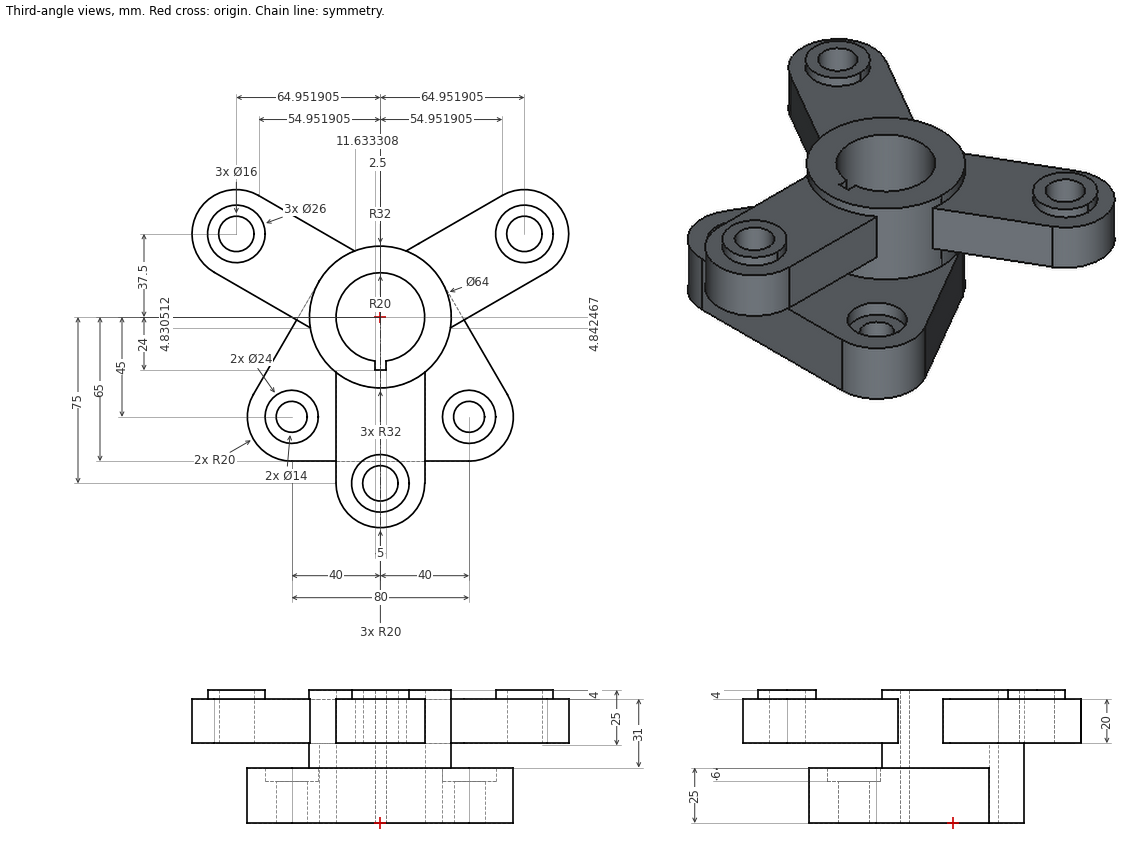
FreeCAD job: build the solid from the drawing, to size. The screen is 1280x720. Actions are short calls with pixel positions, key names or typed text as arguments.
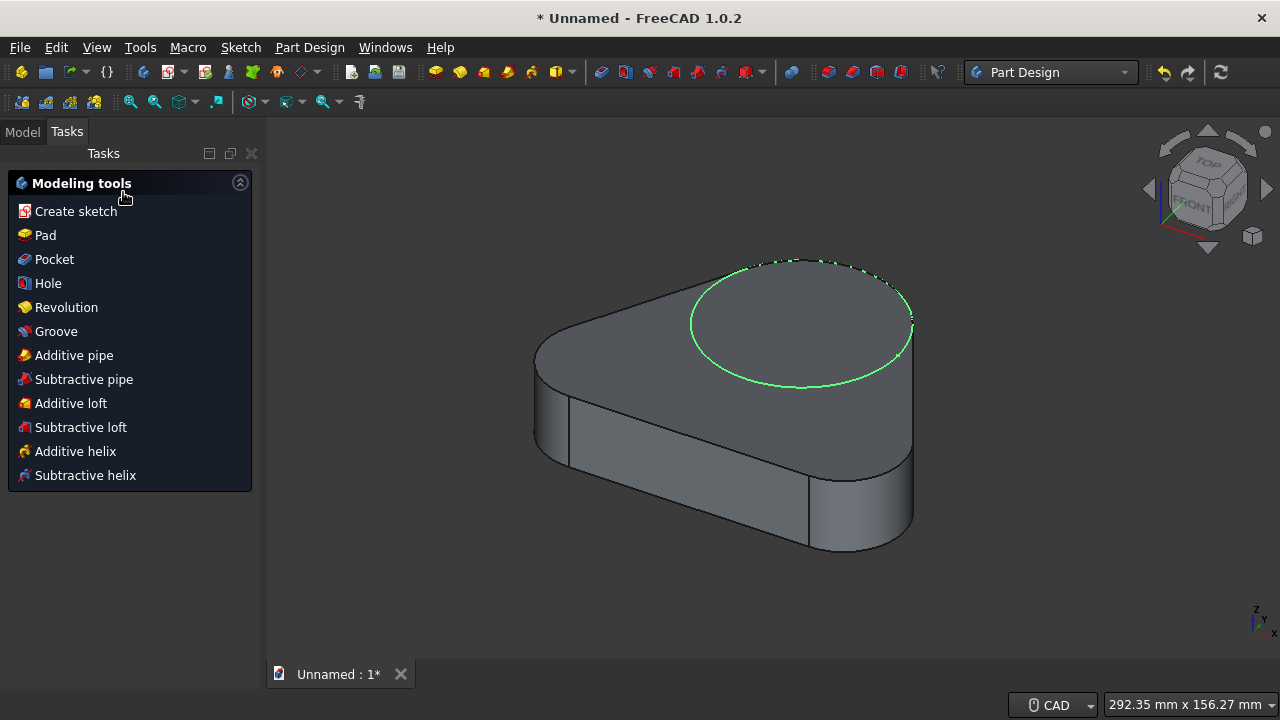
click(436, 72)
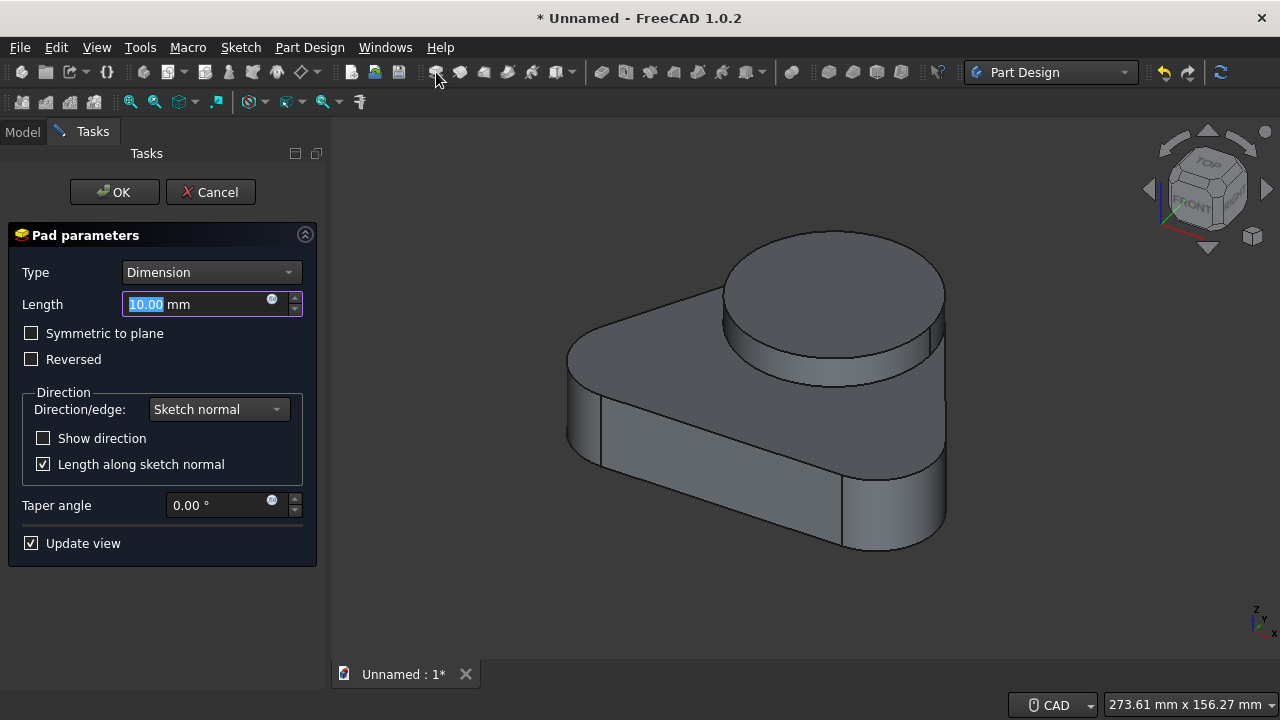
text(31)
key(Tab)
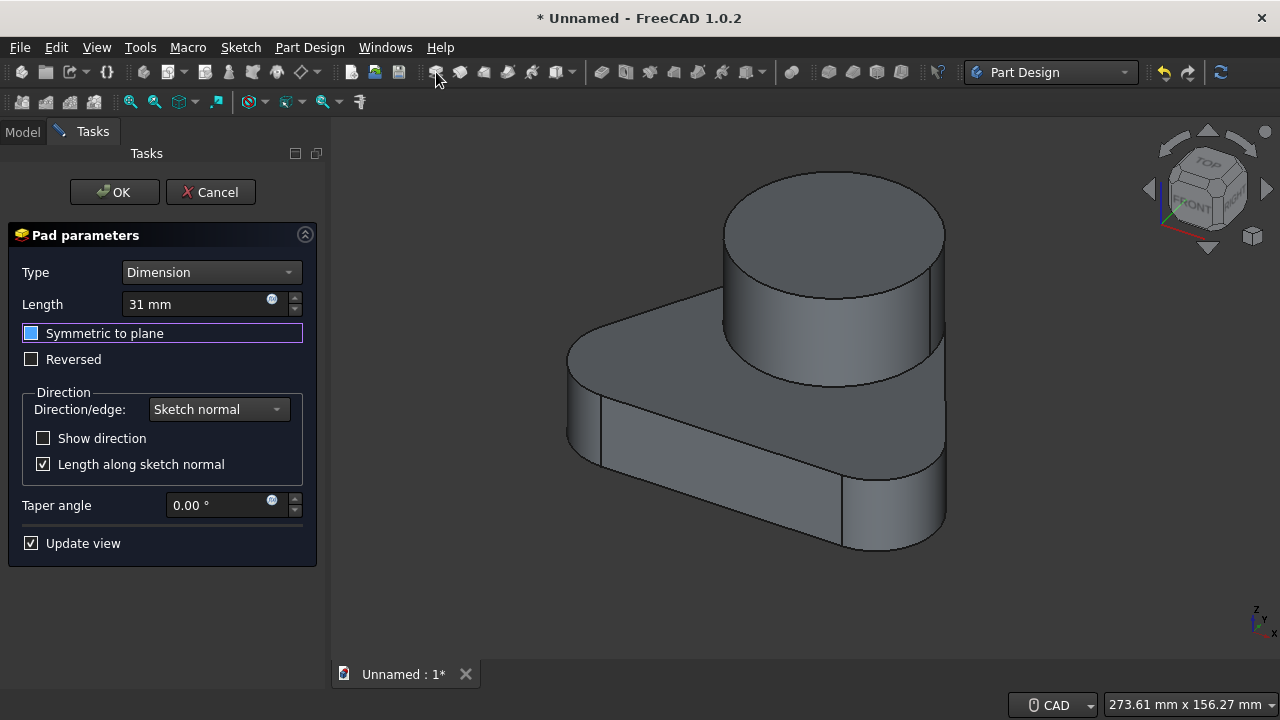
click(115, 192)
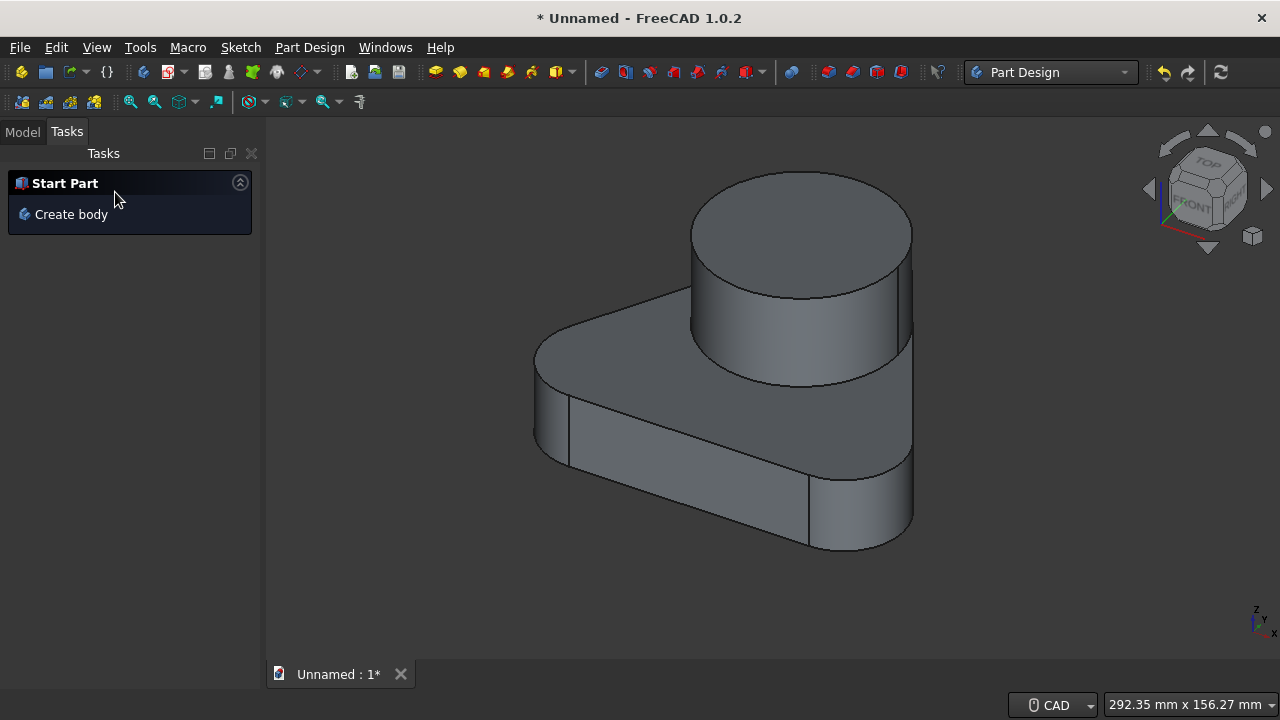
click(23, 131)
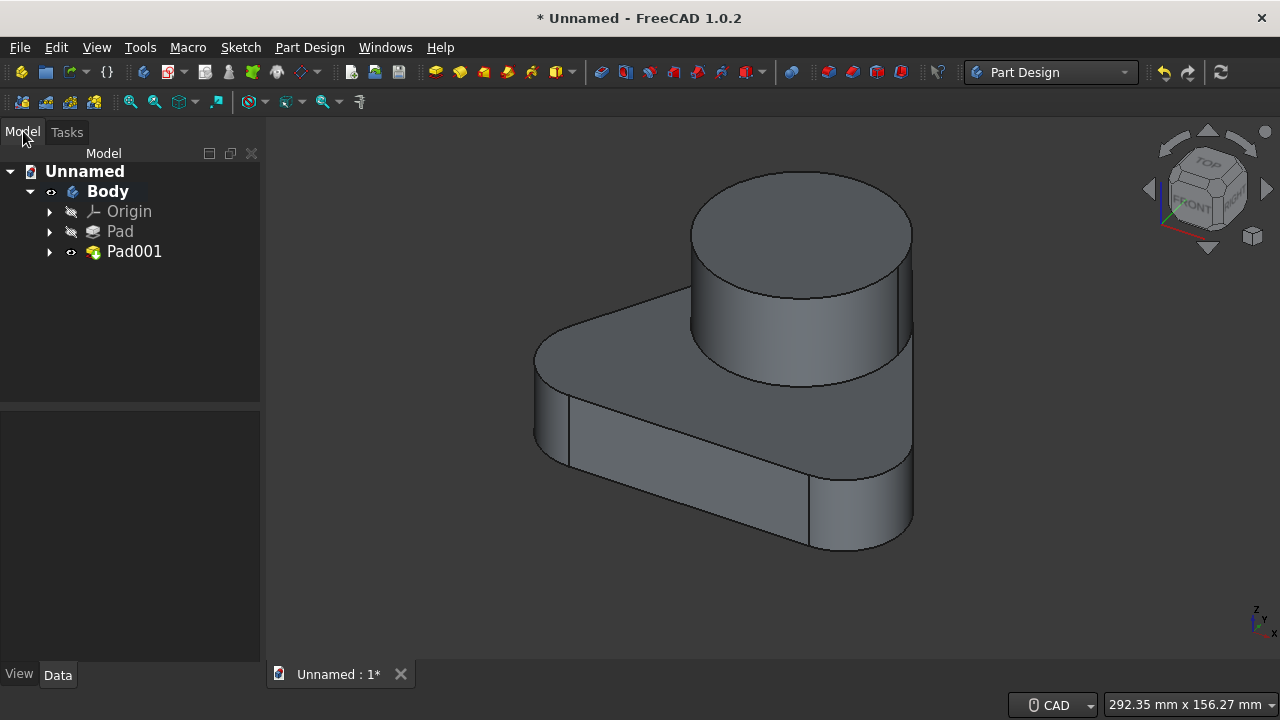
click(50, 212)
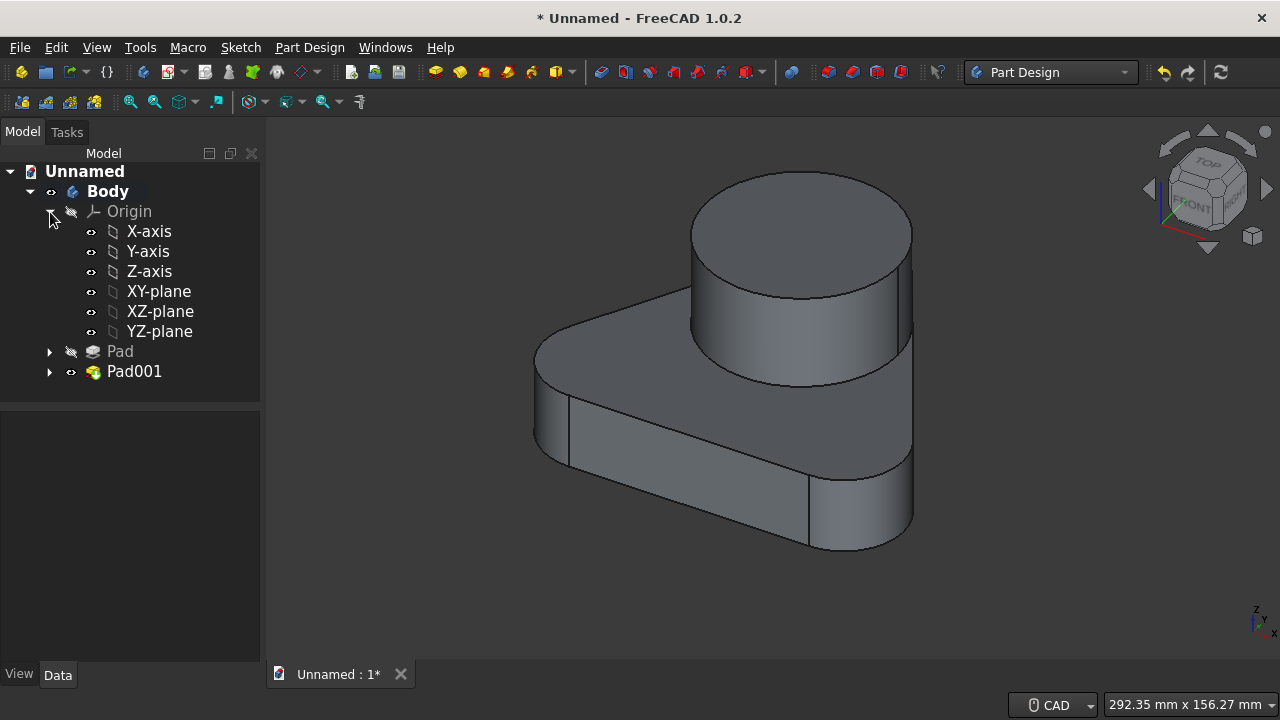
click(136, 292)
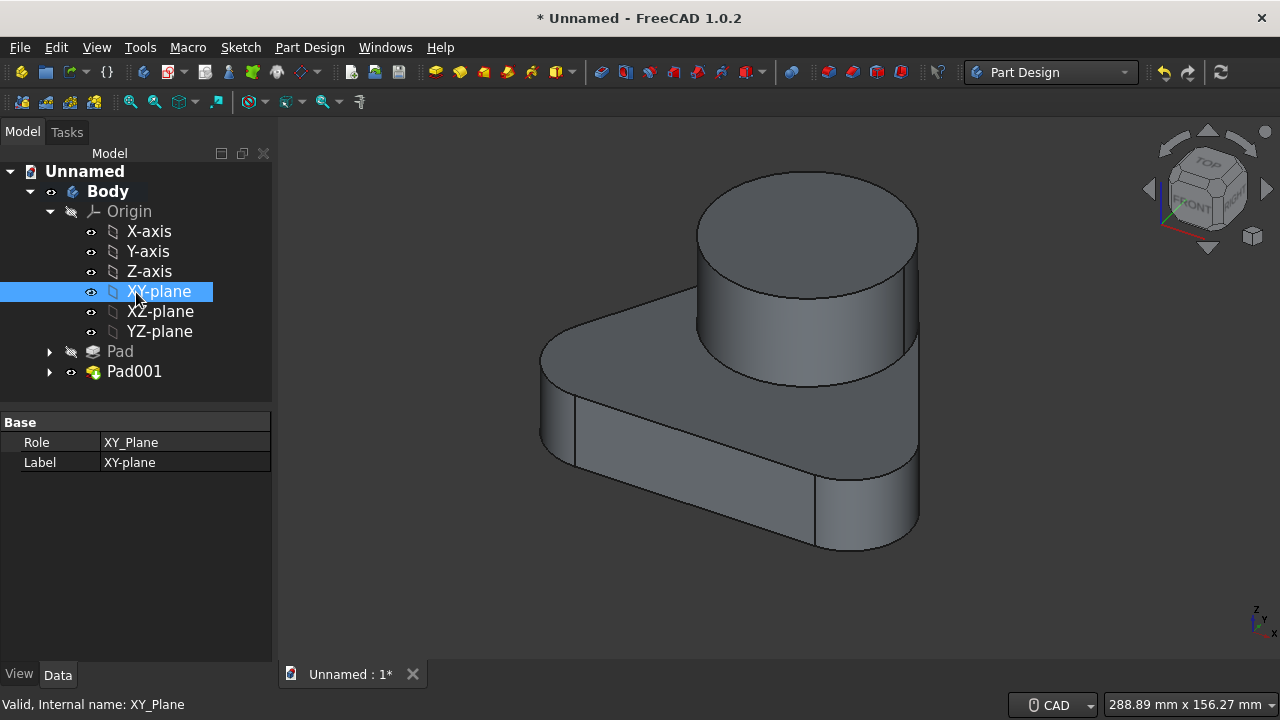
click(302, 72)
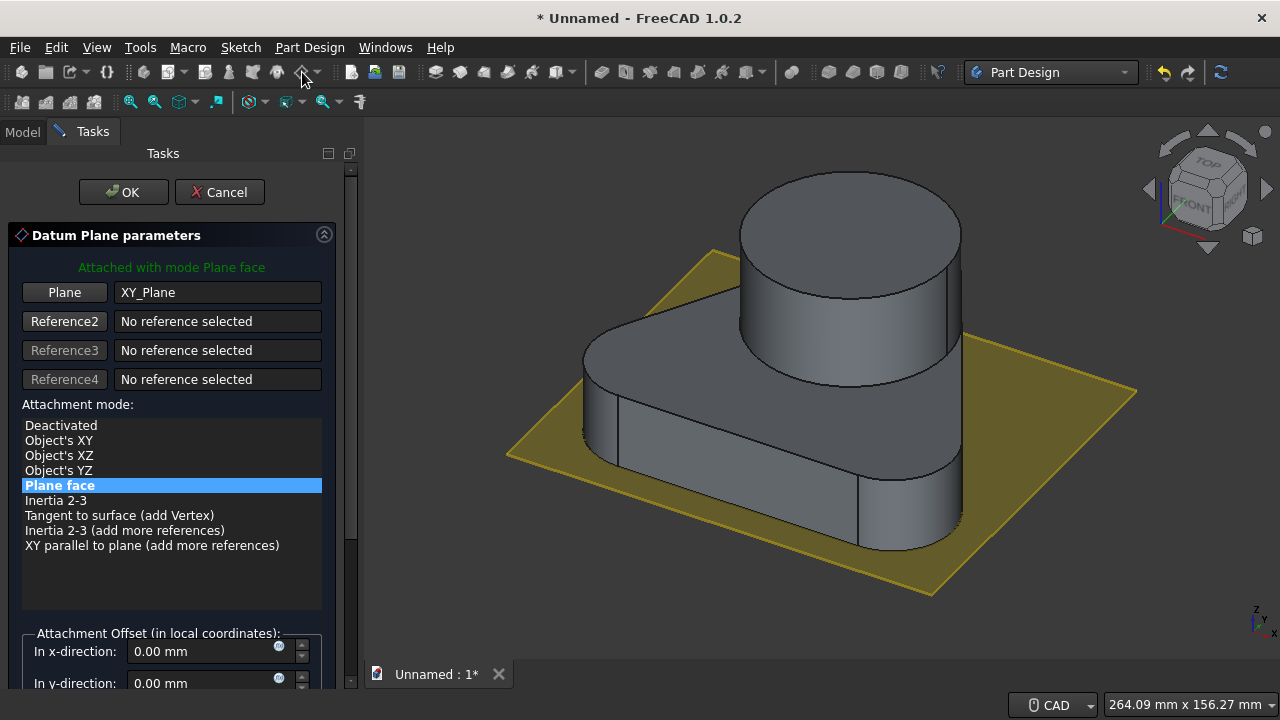
scroll(351, 426, down, 2)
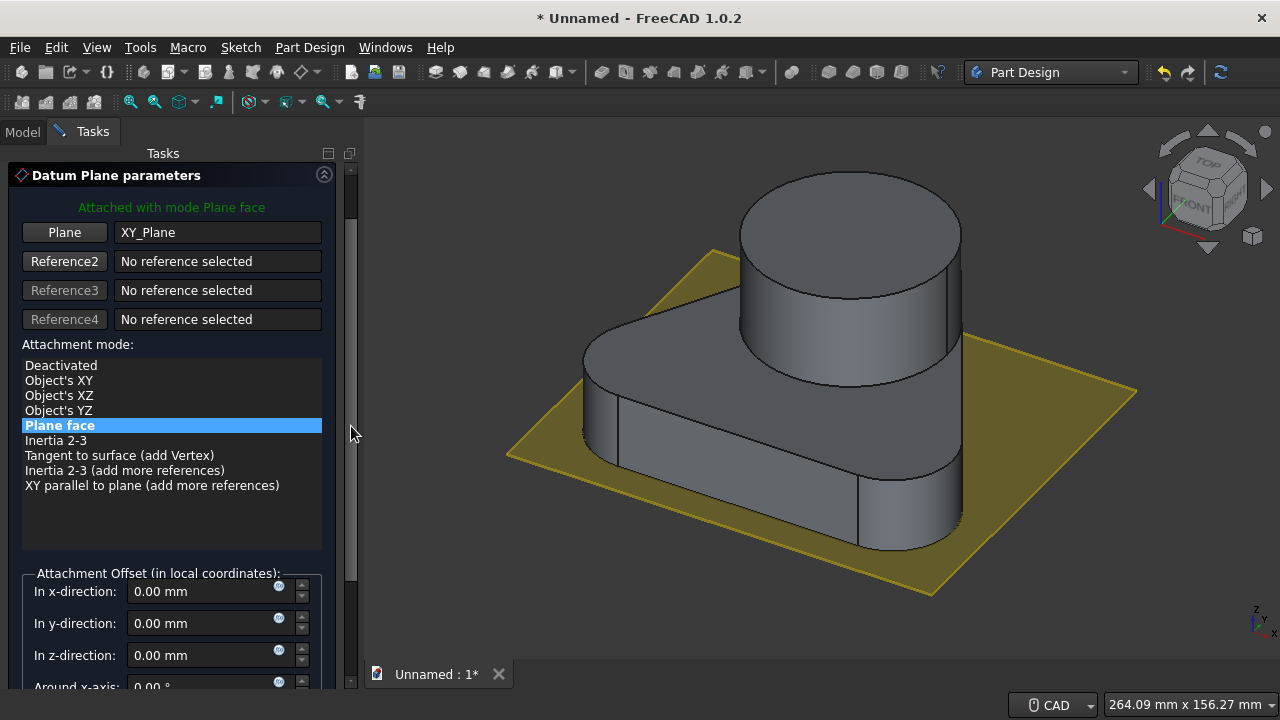
triple_click(210, 595)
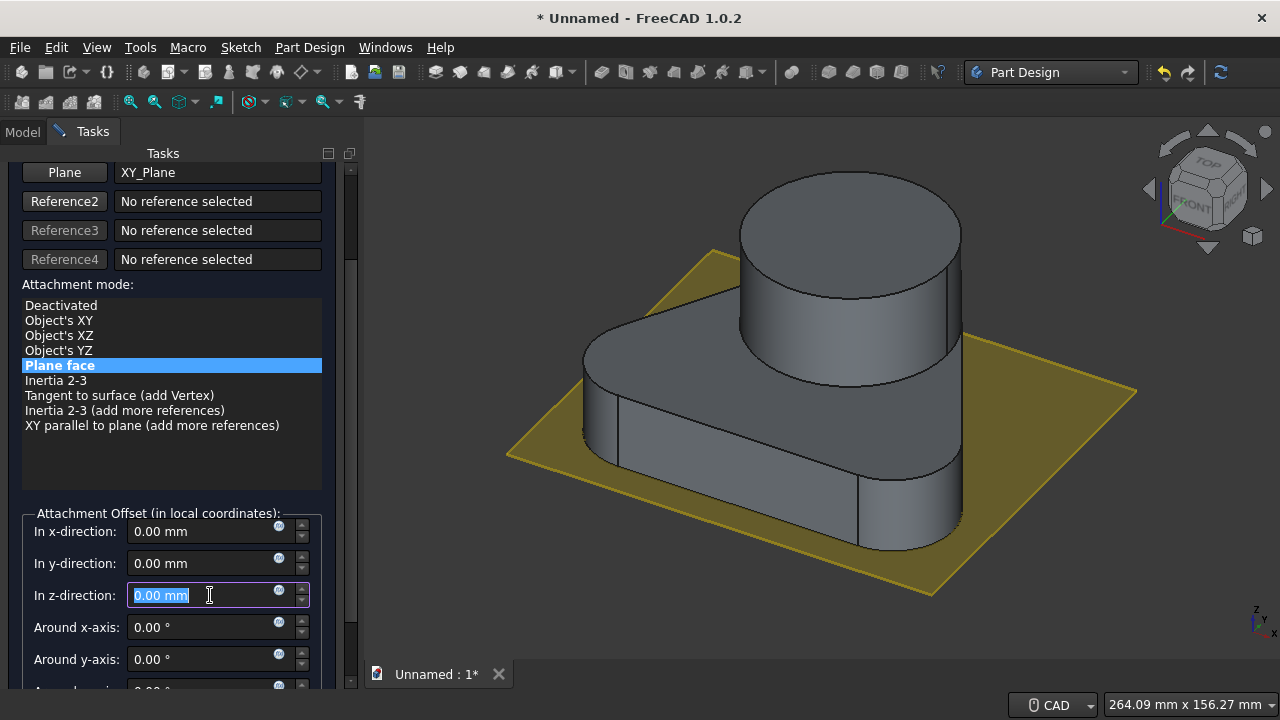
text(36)
key(Tab)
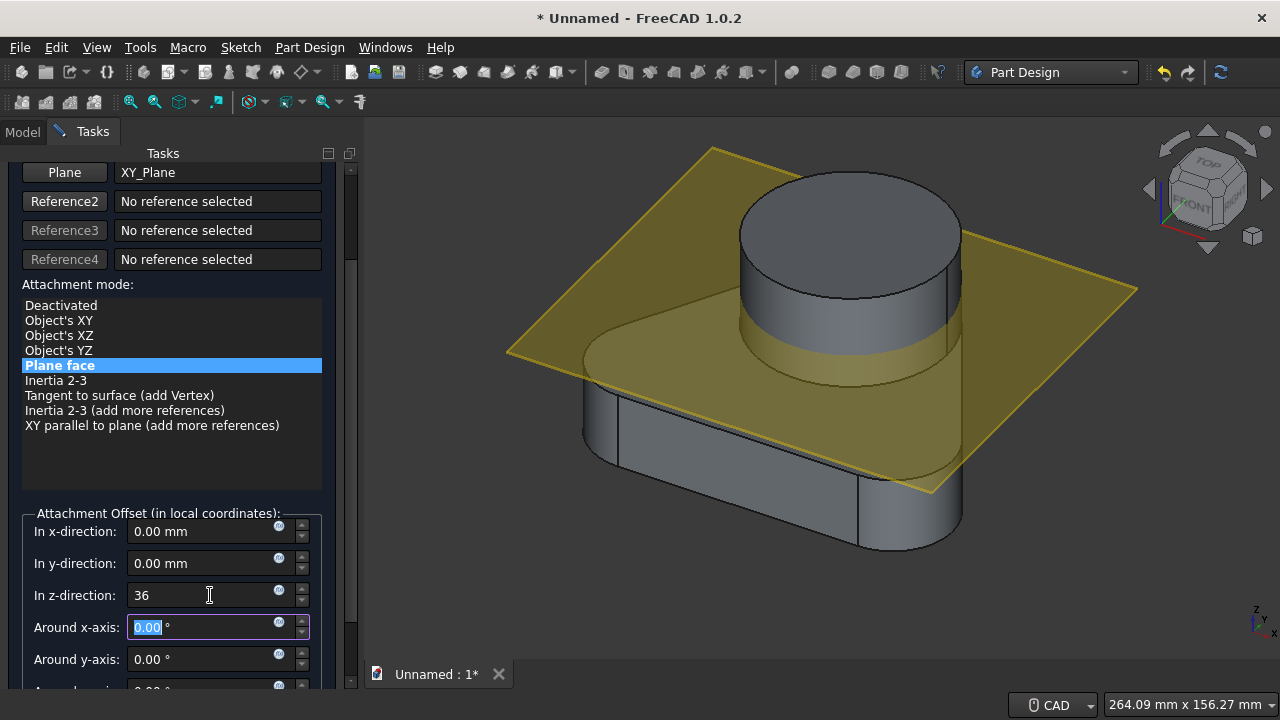
scroll(351, 426, up, 3)